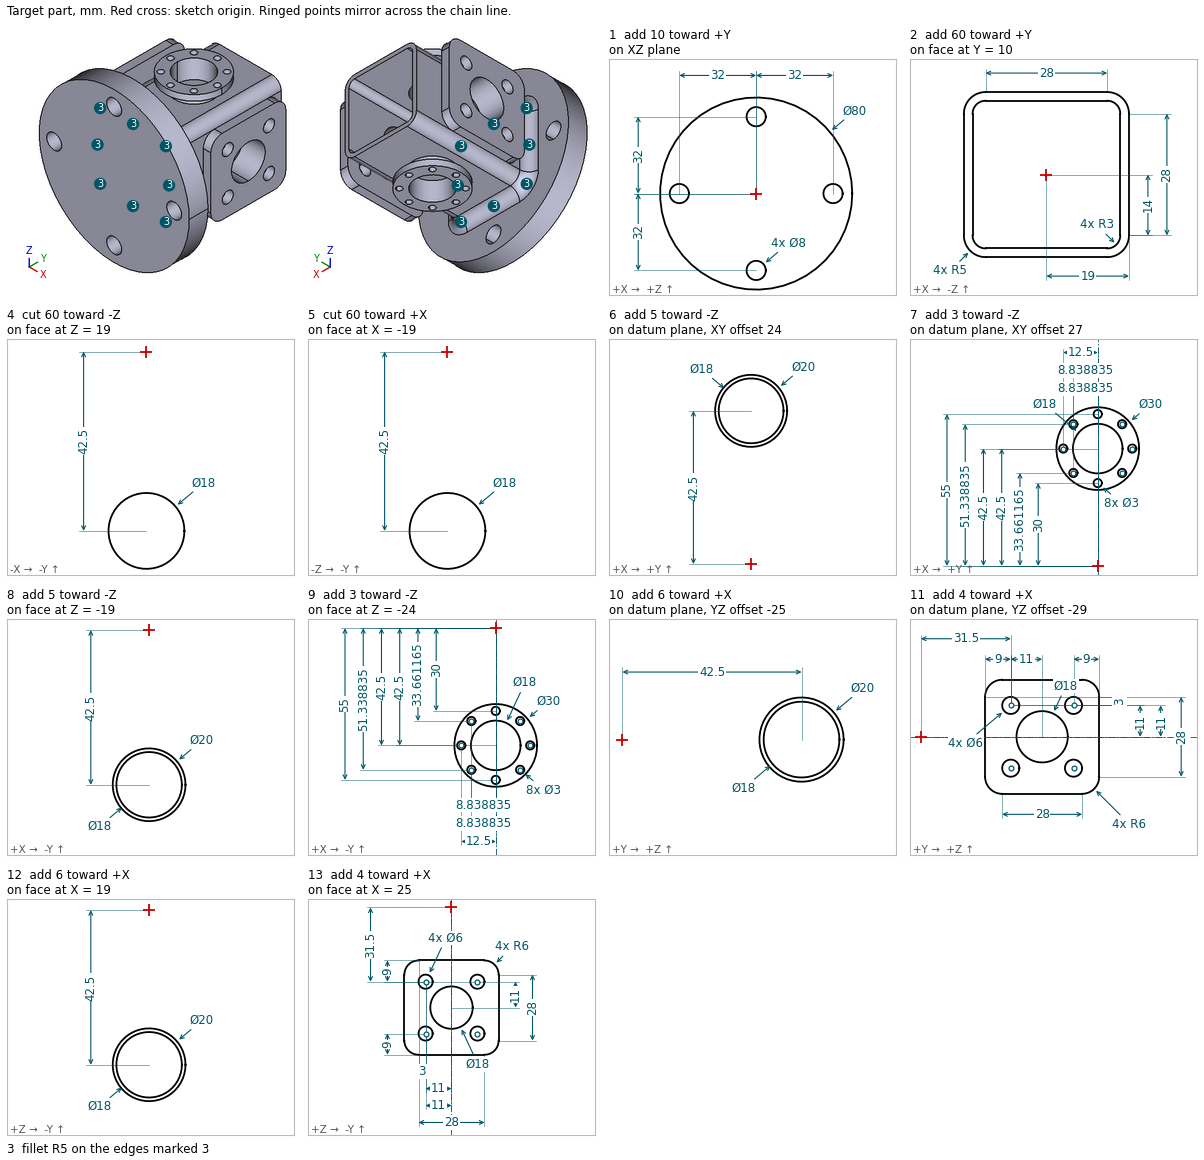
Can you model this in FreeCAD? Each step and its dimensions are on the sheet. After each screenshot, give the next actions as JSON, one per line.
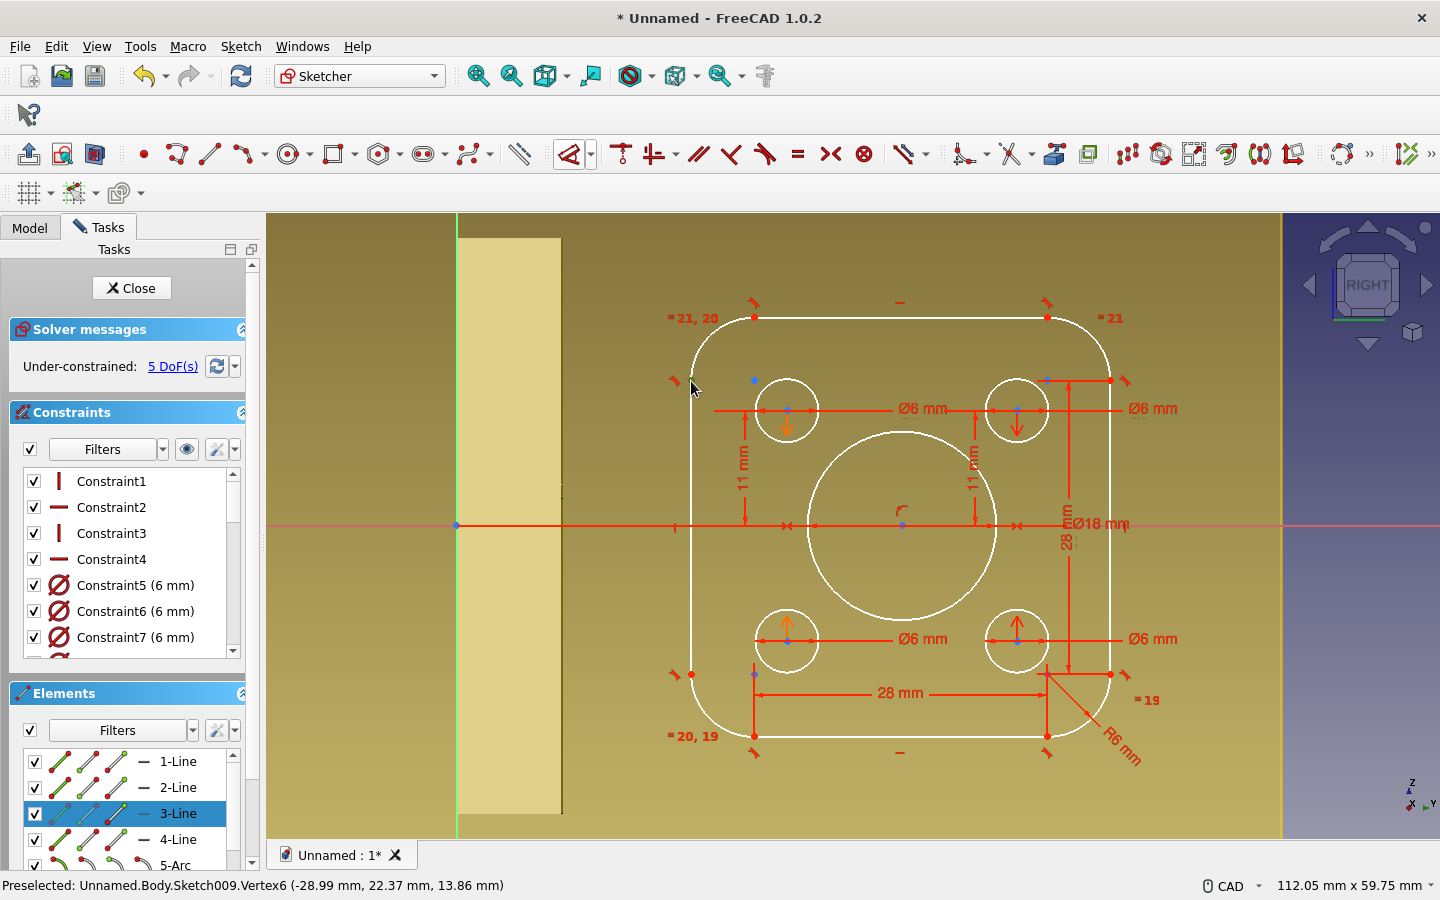
{"action": "left_click", "coordinate": [787, 411]}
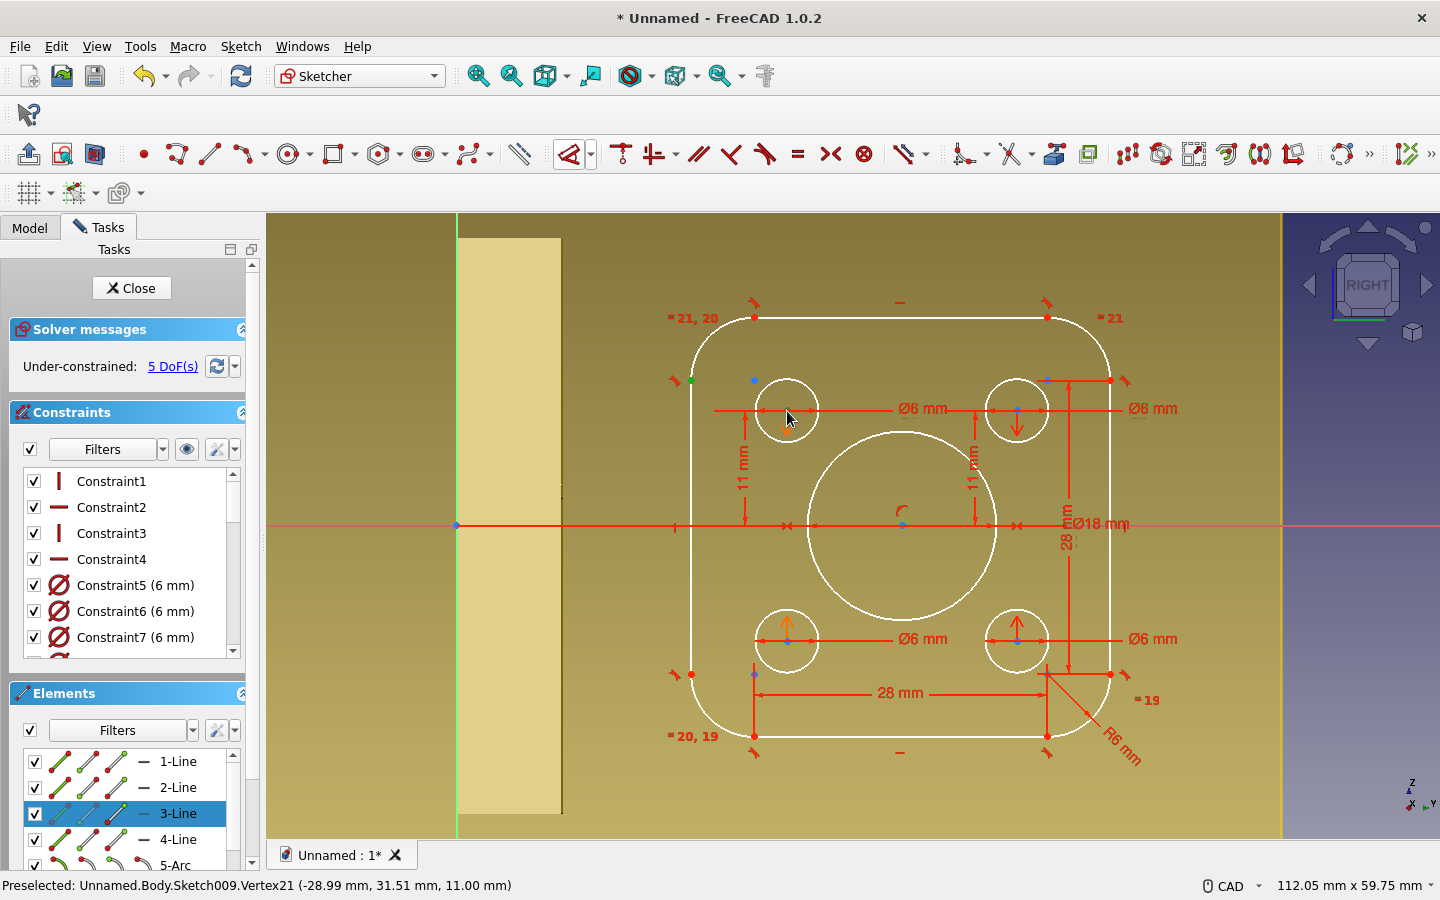
{"action": "key", "text": "l"}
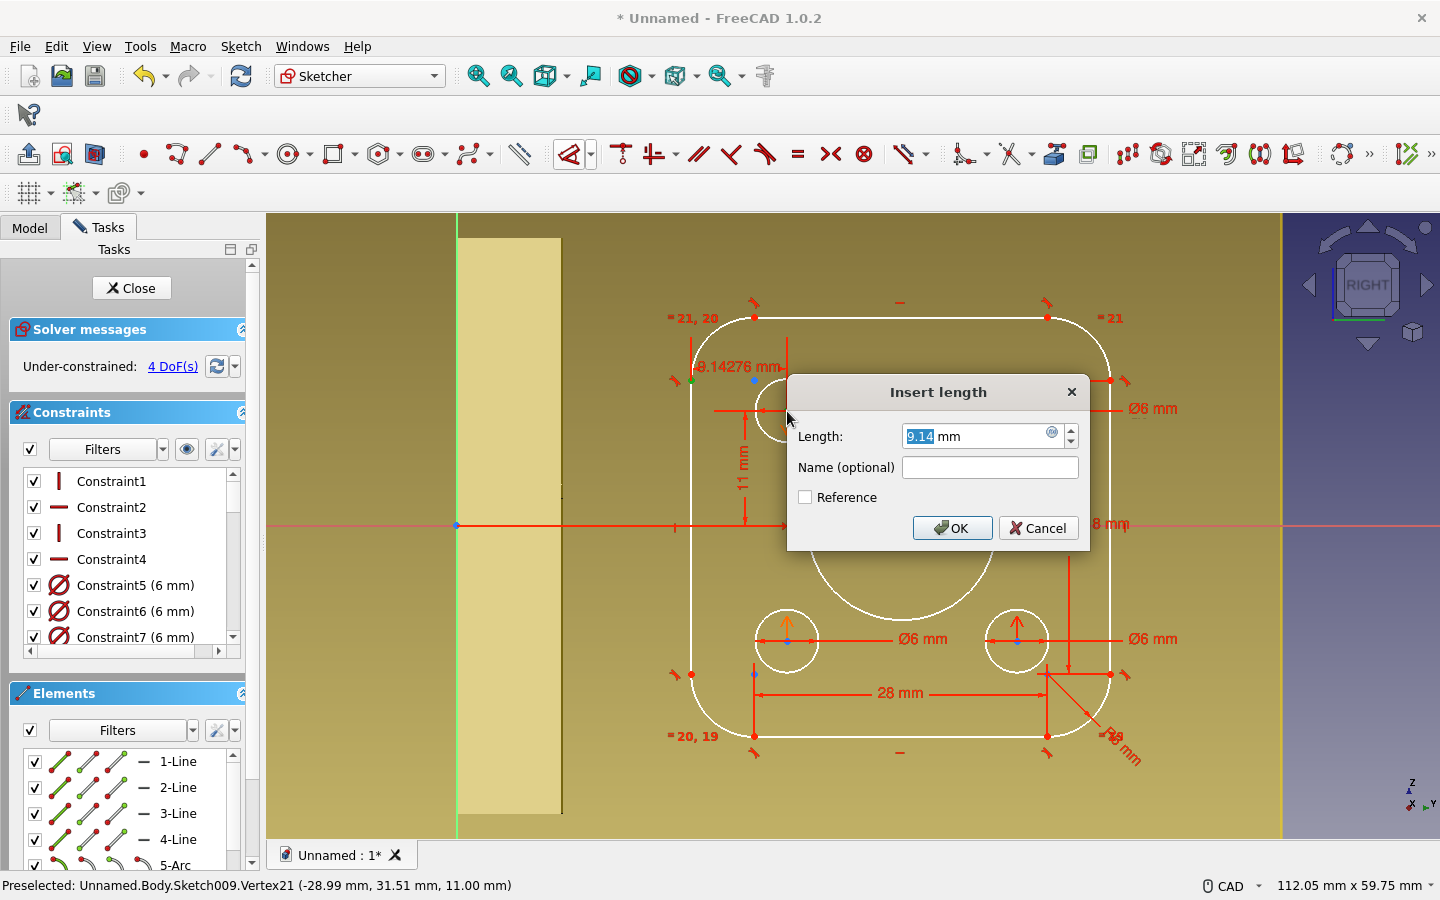
{"action": "type", "text": "9"}
{"action": "key", "text": "Return"}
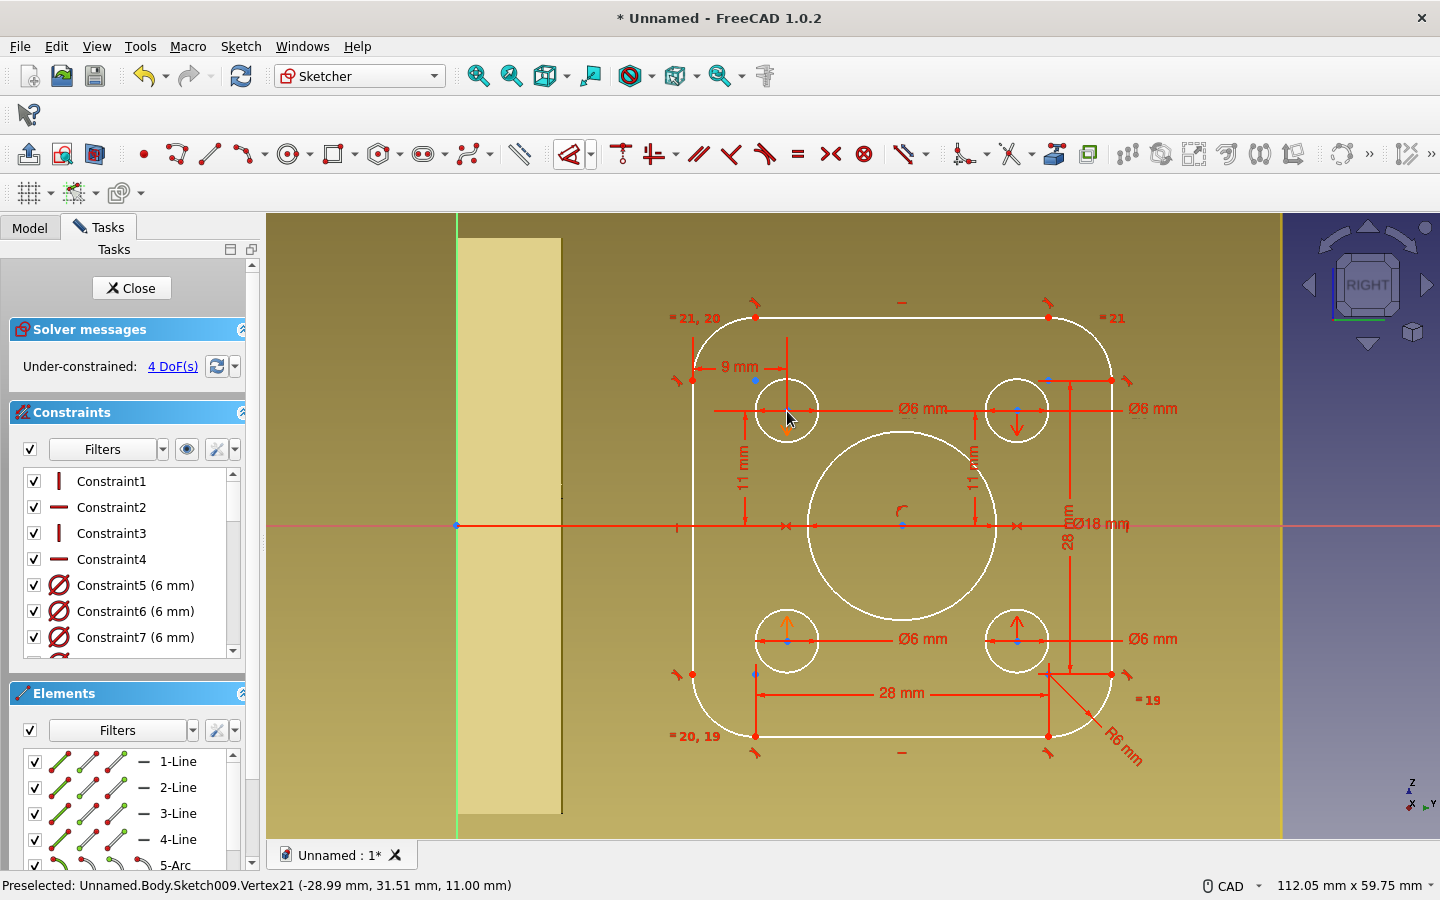
{"action": "scroll", "coordinate": [693, 381], "scroll_direction": "up", "scroll_amount": 2}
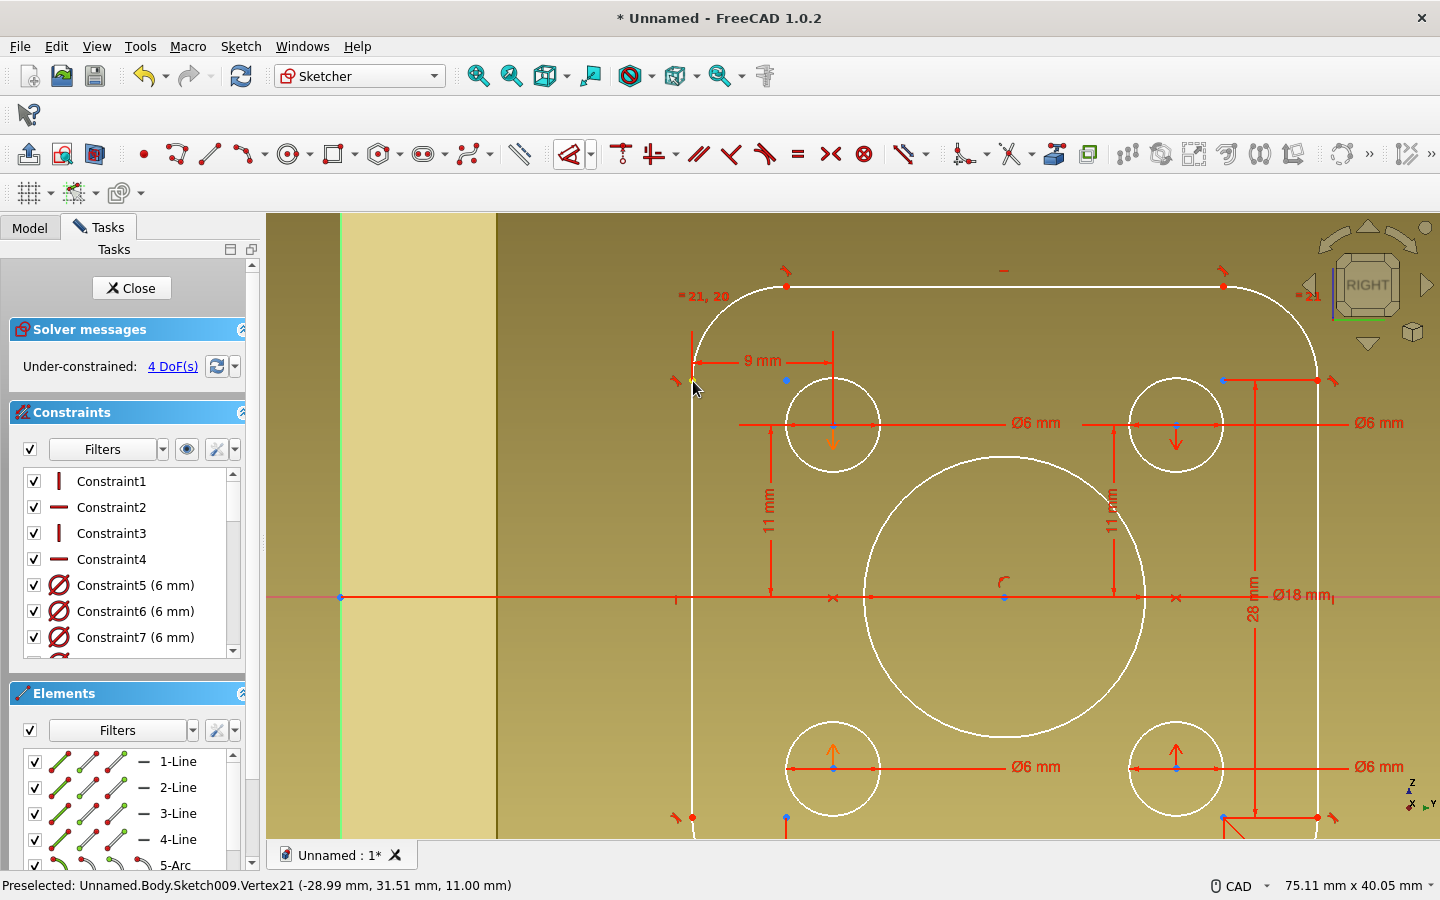
{"action": "left_click", "coordinate": [692, 380]}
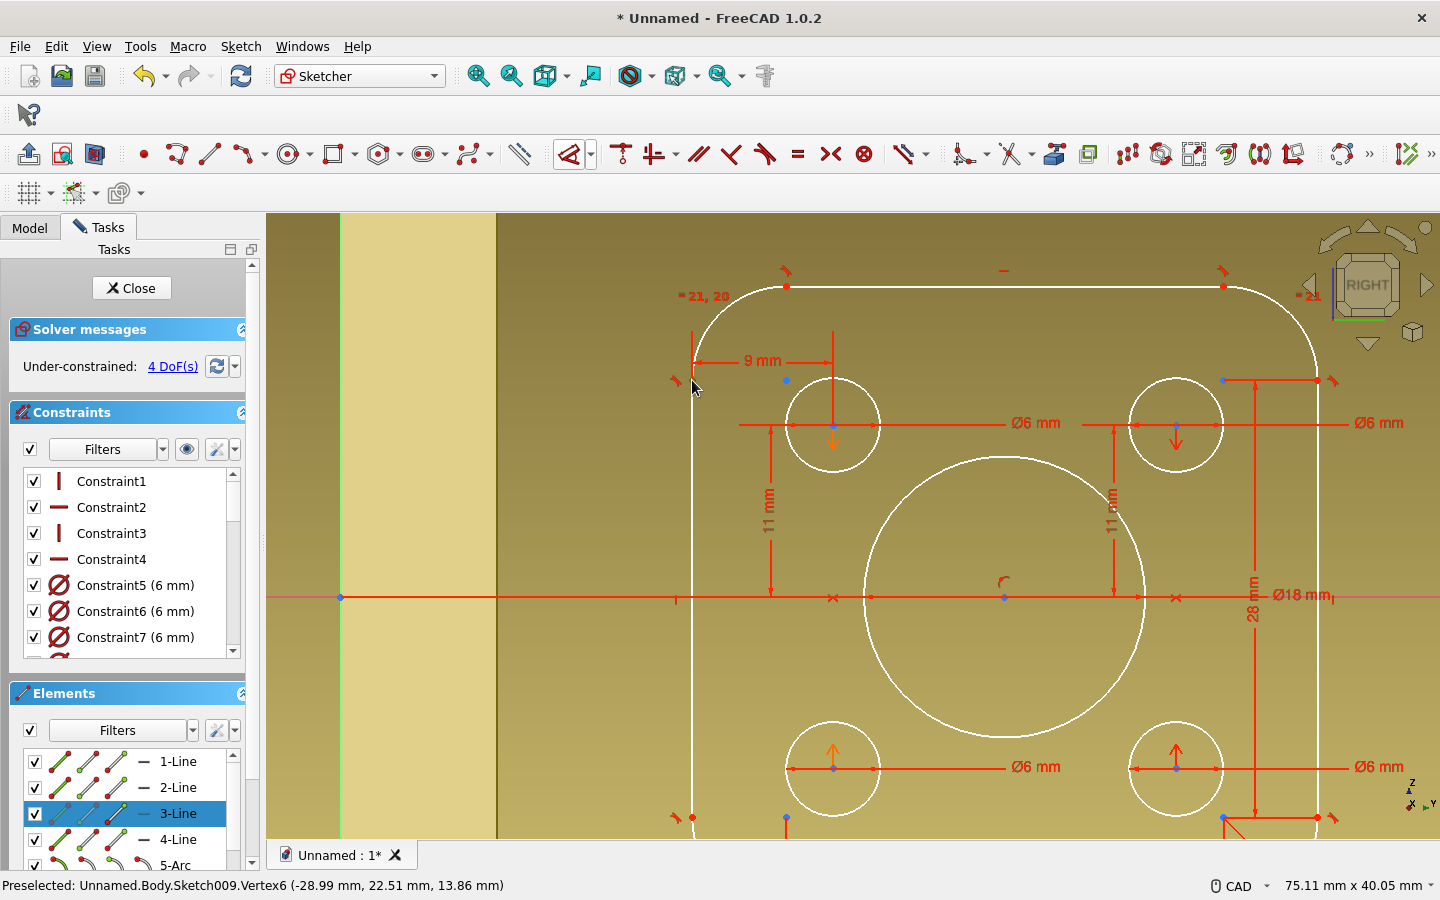
{"action": "left_click", "coordinate": [833, 425]}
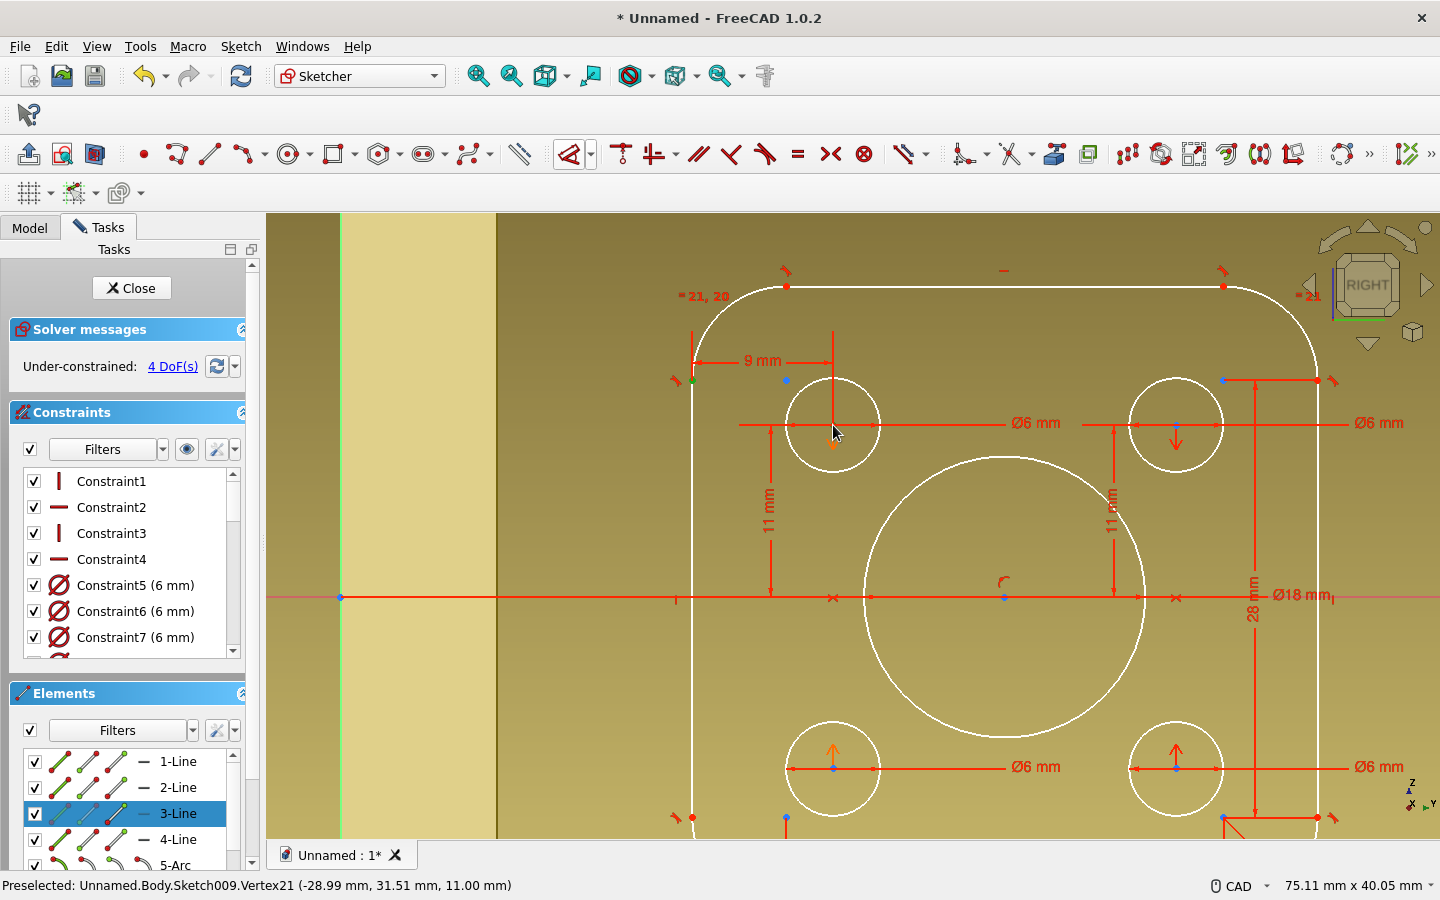
{"action": "left_click", "coordinate": [590, 154]}